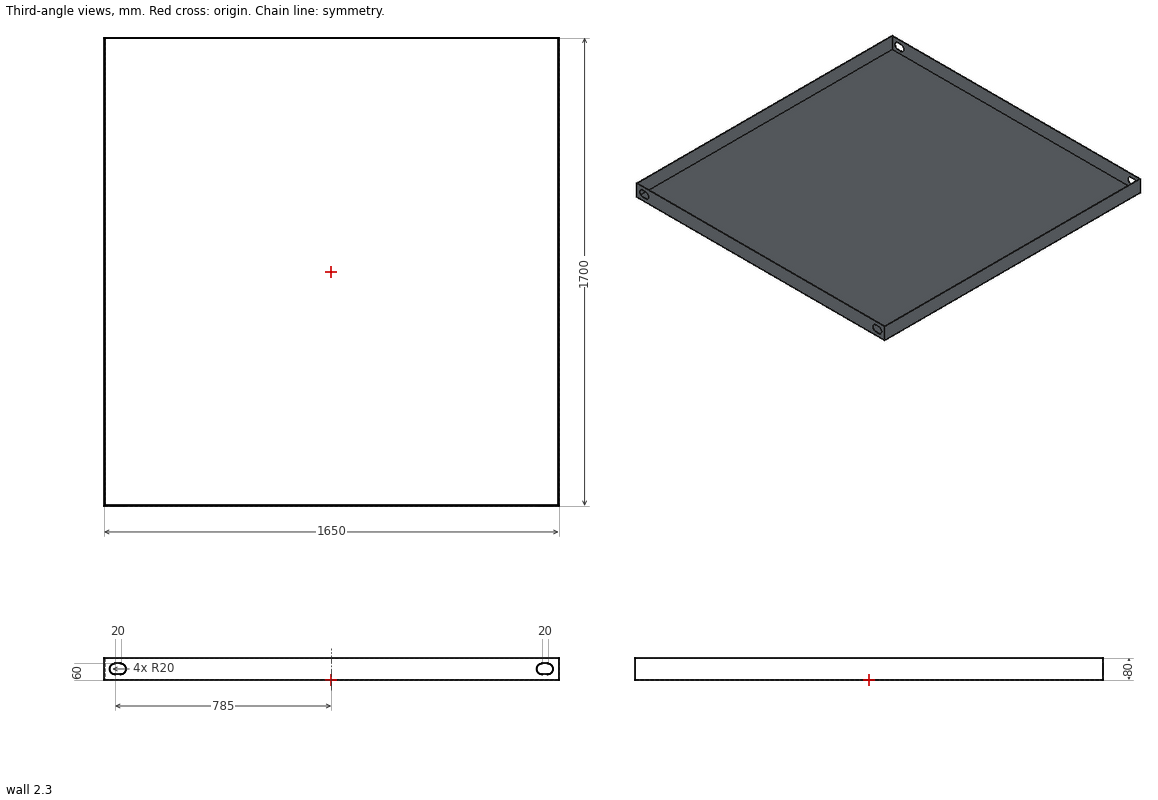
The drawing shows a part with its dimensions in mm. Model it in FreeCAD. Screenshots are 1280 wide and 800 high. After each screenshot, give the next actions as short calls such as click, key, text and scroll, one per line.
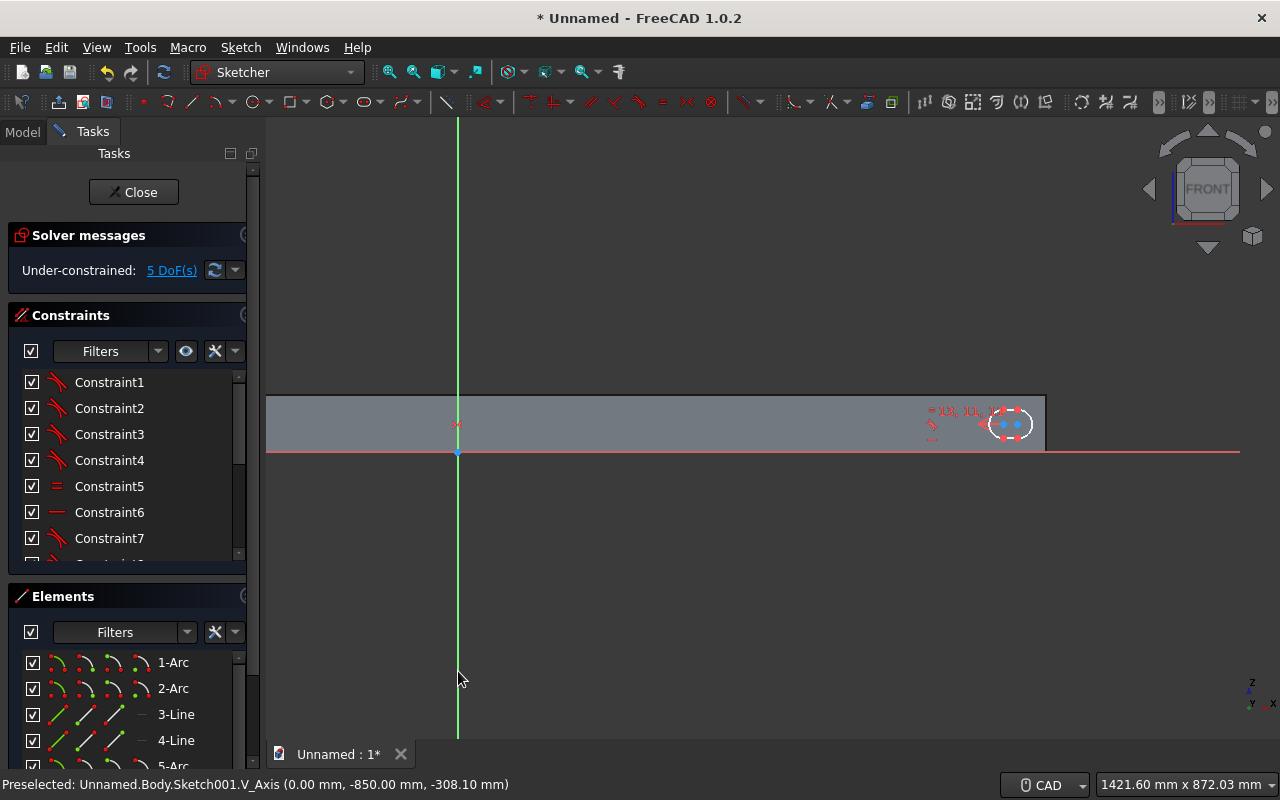
scroll(1005, 425, down, 3)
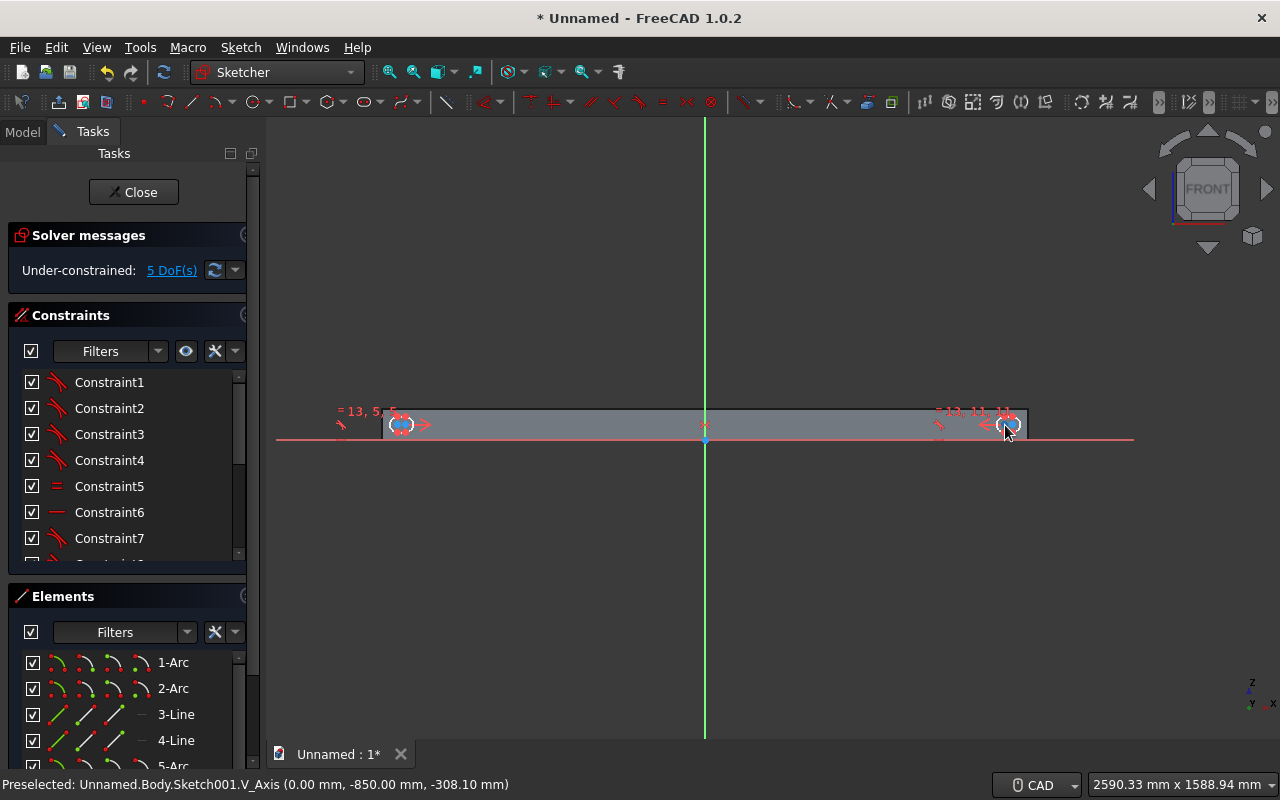
scroll(391, 420, up, 9)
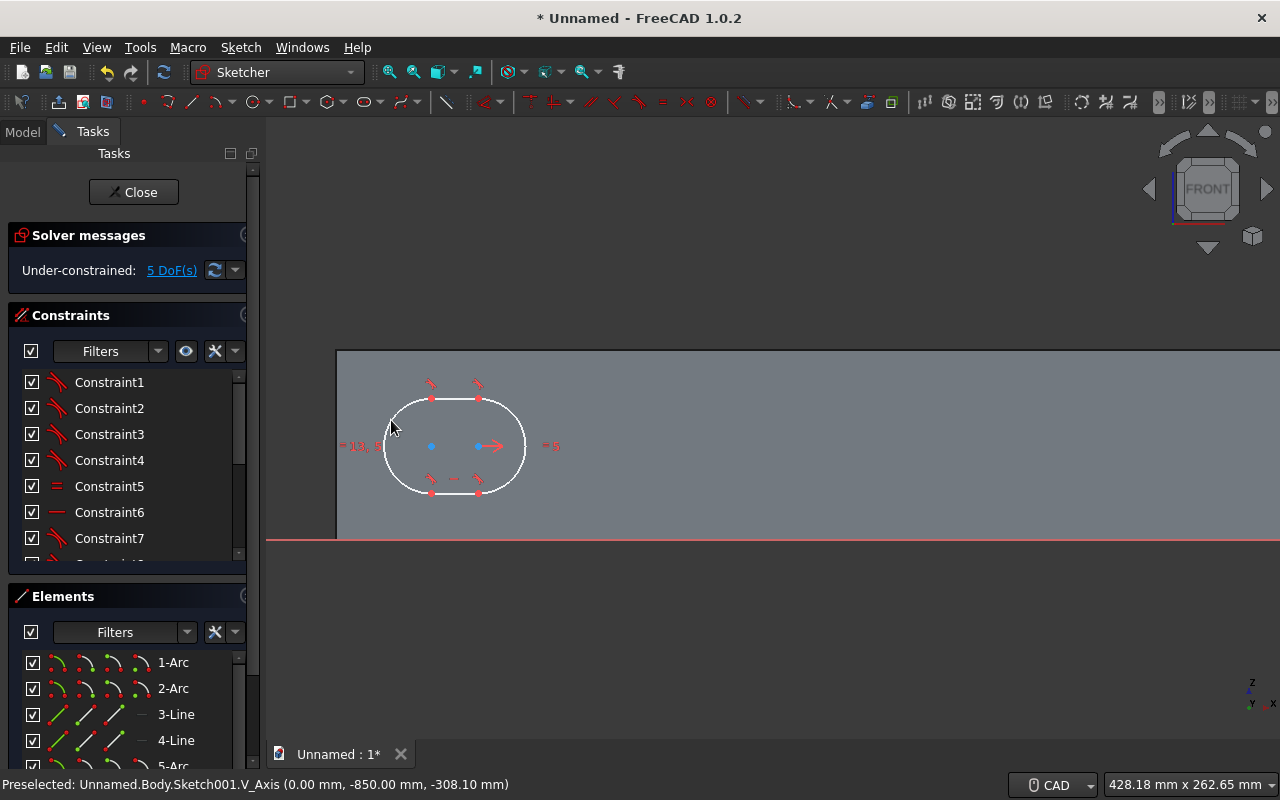
click(393, 418)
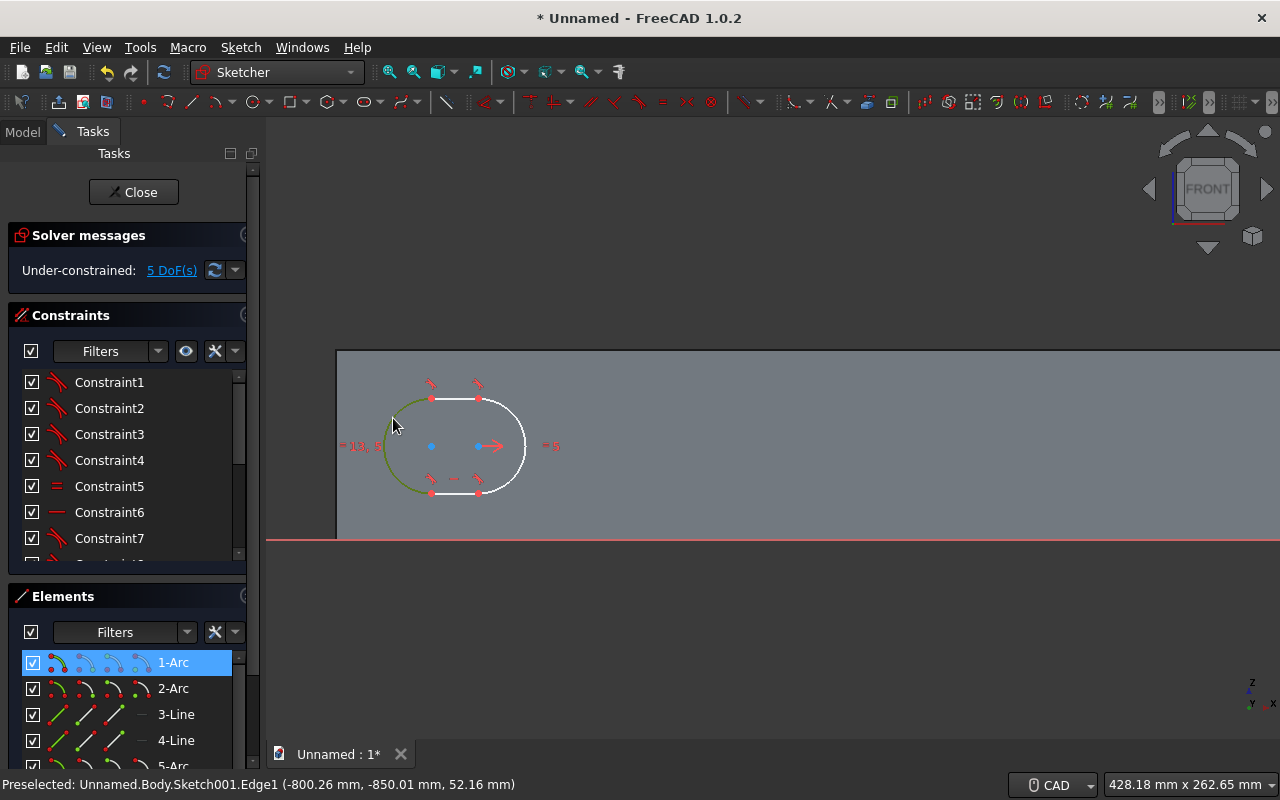
click(502, 102)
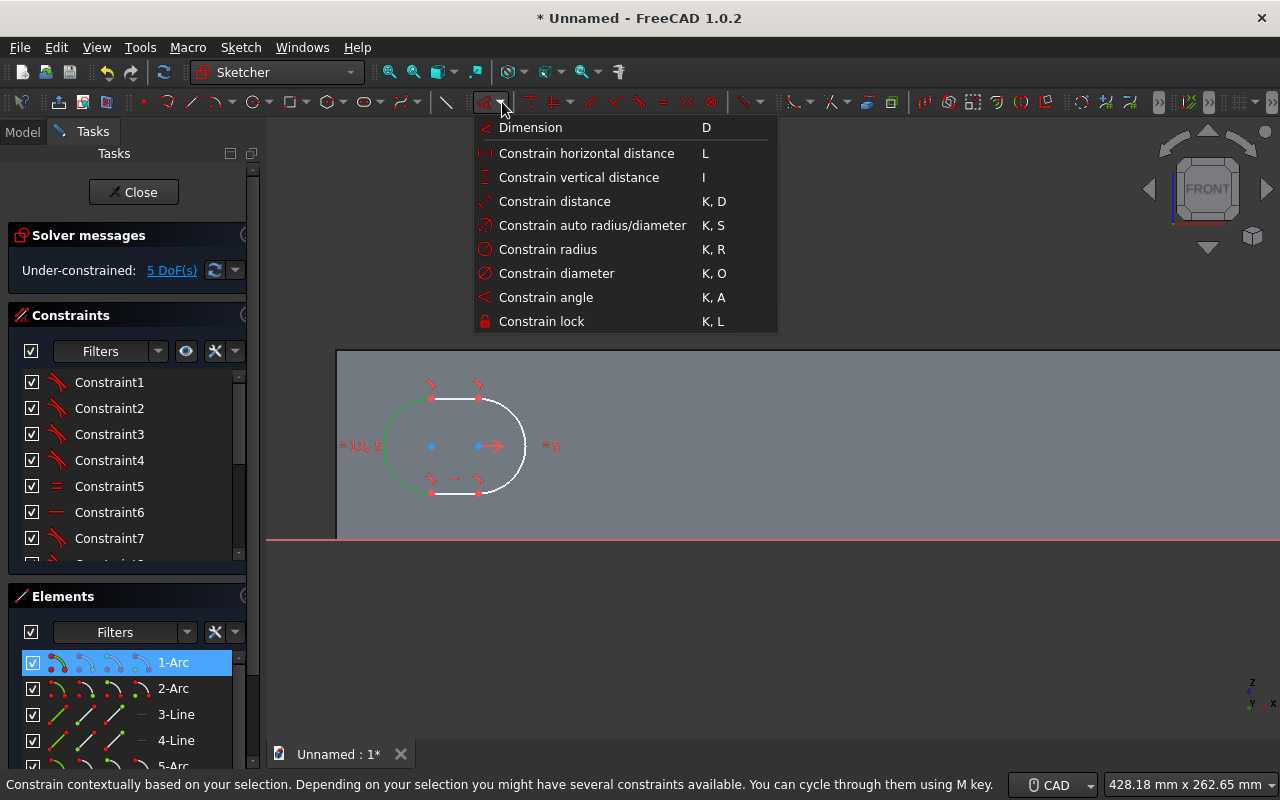
click(626, 249)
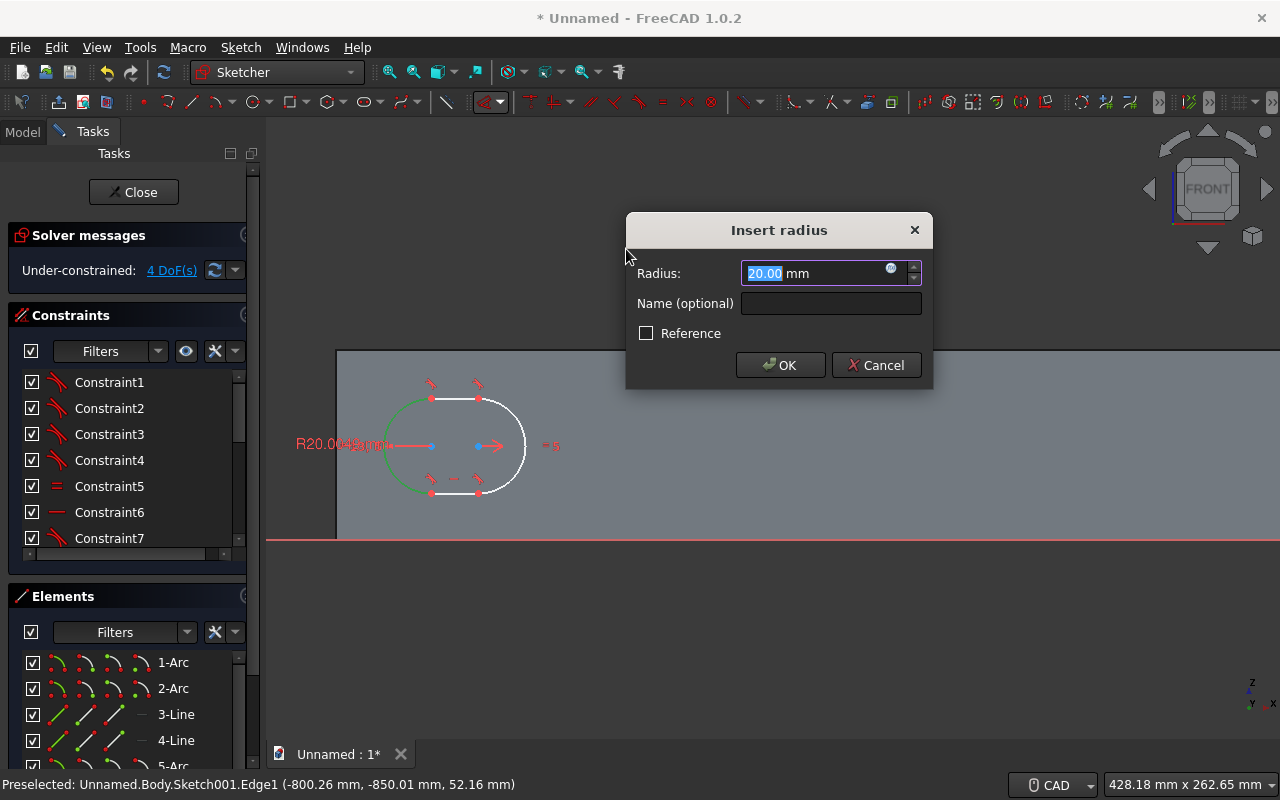
text(20)
key(Return)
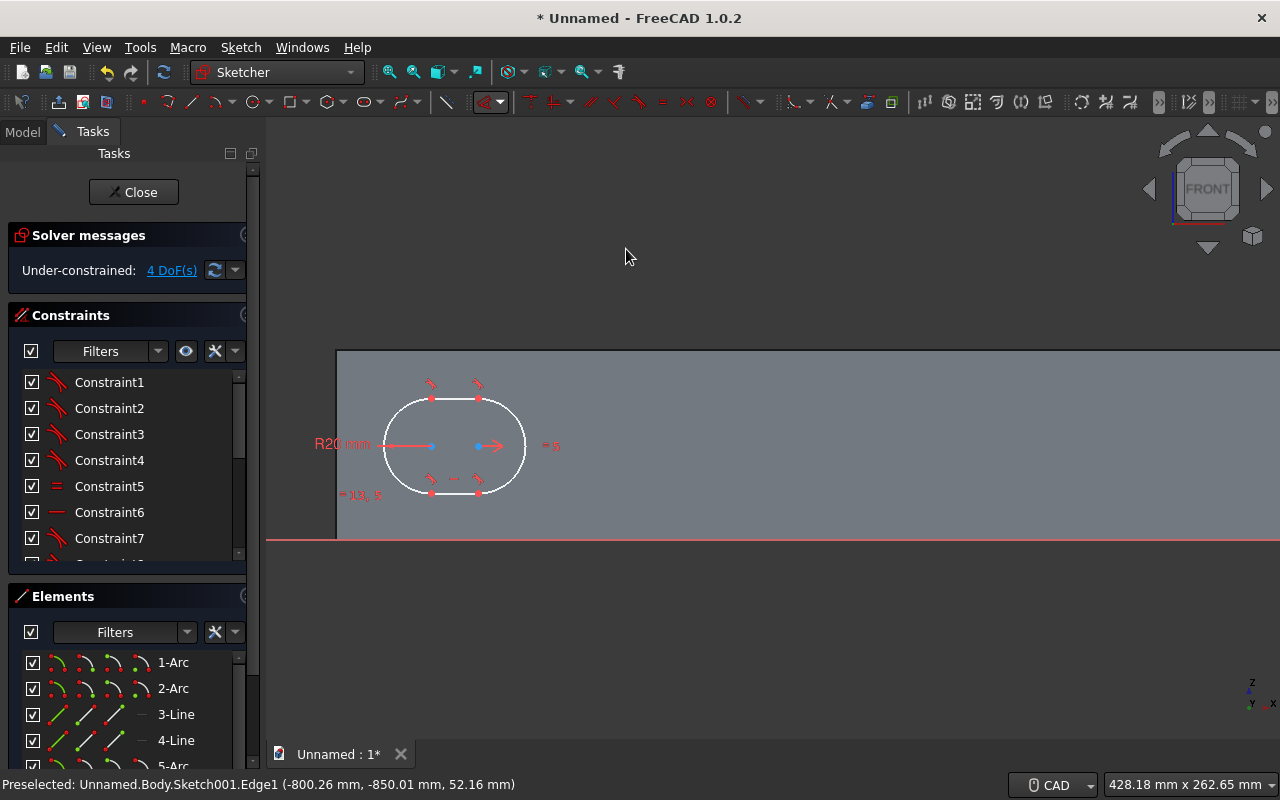
click(445, 399)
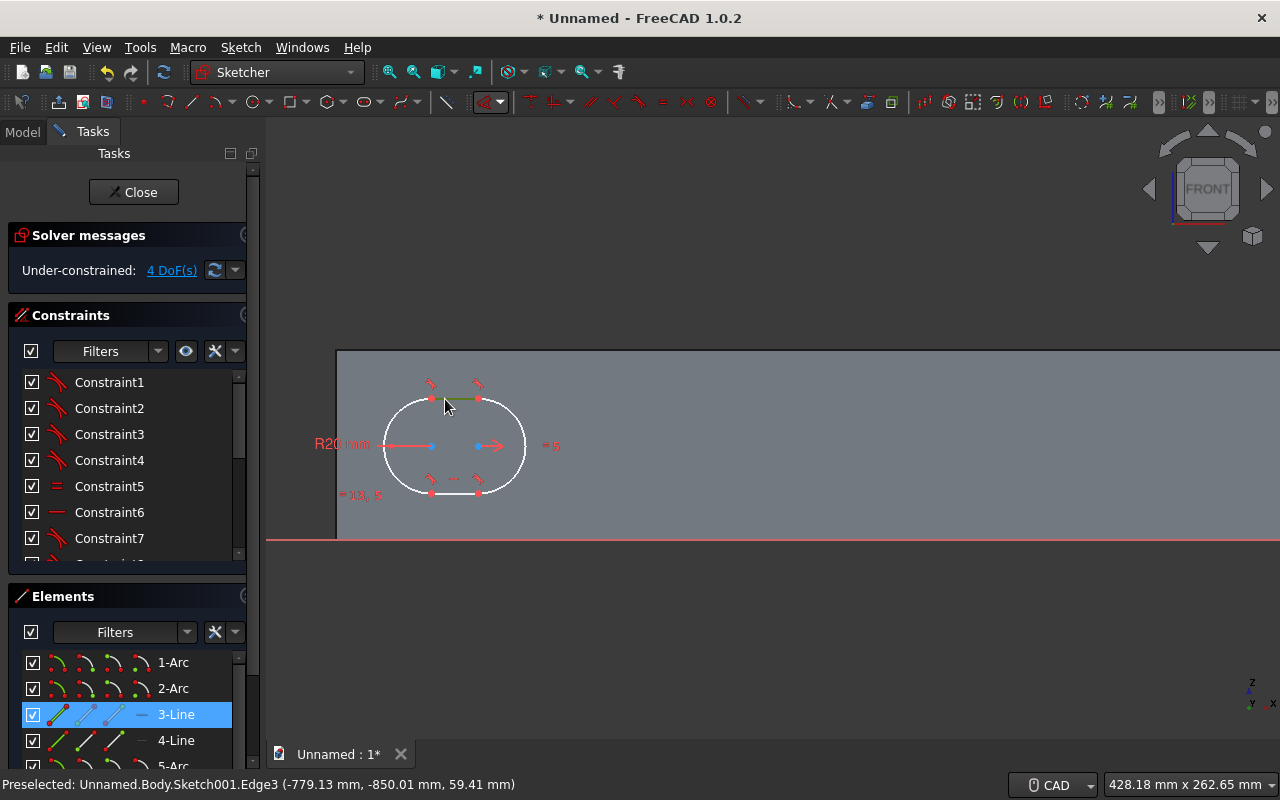
key(l)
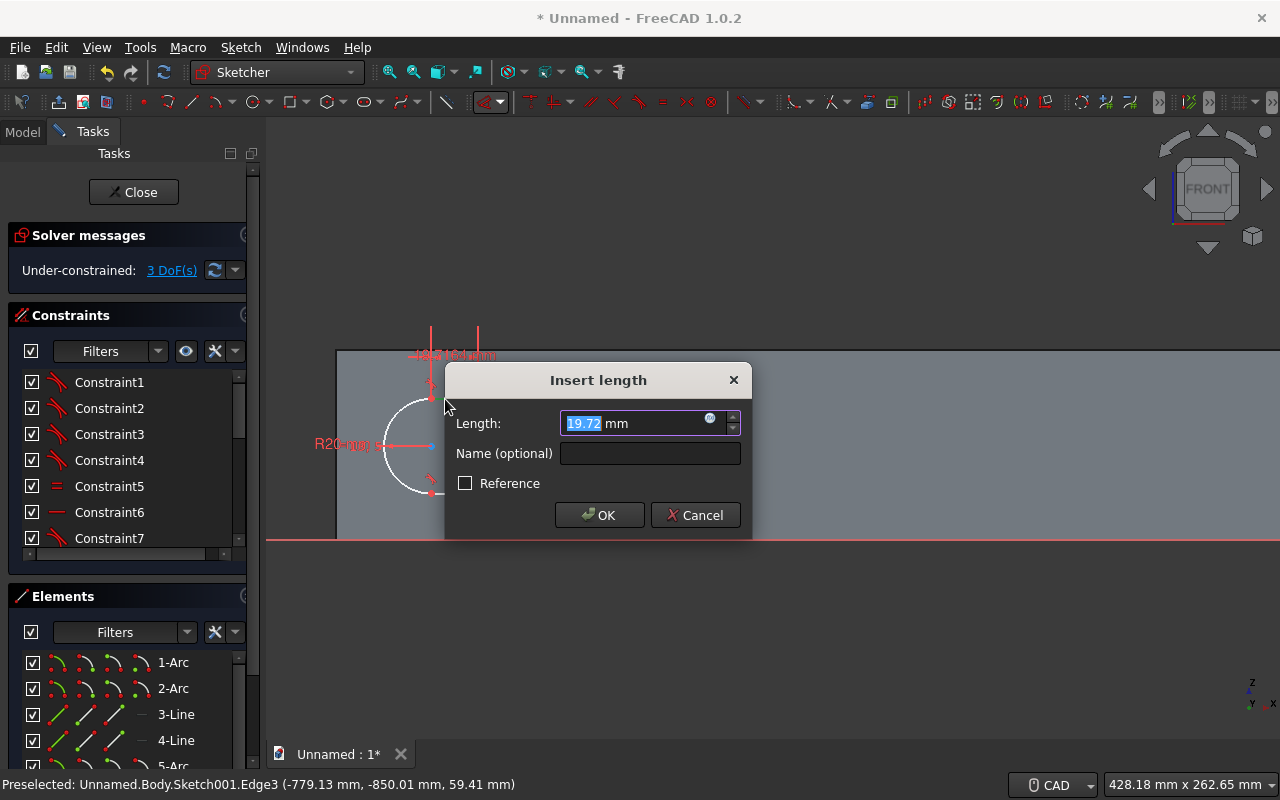
text(20)
key(Return)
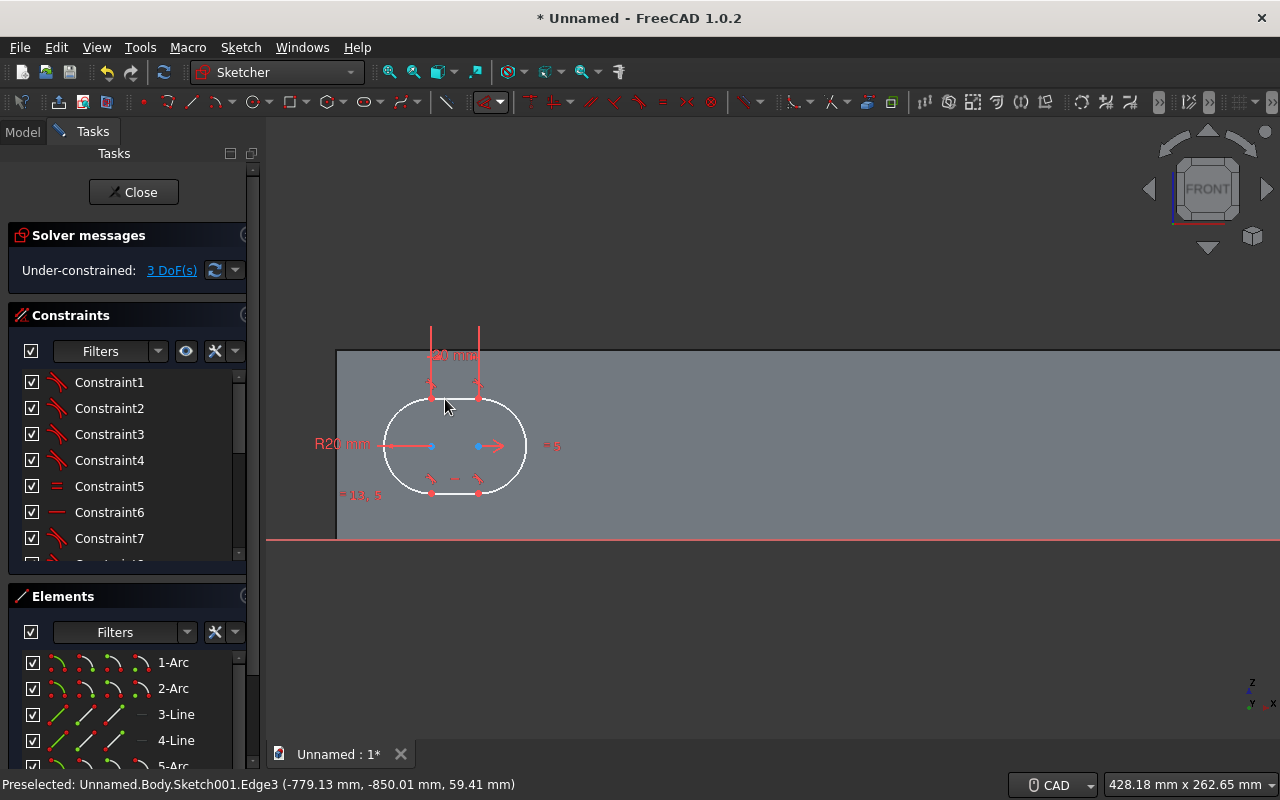
scroll(390, 420, down, 9)